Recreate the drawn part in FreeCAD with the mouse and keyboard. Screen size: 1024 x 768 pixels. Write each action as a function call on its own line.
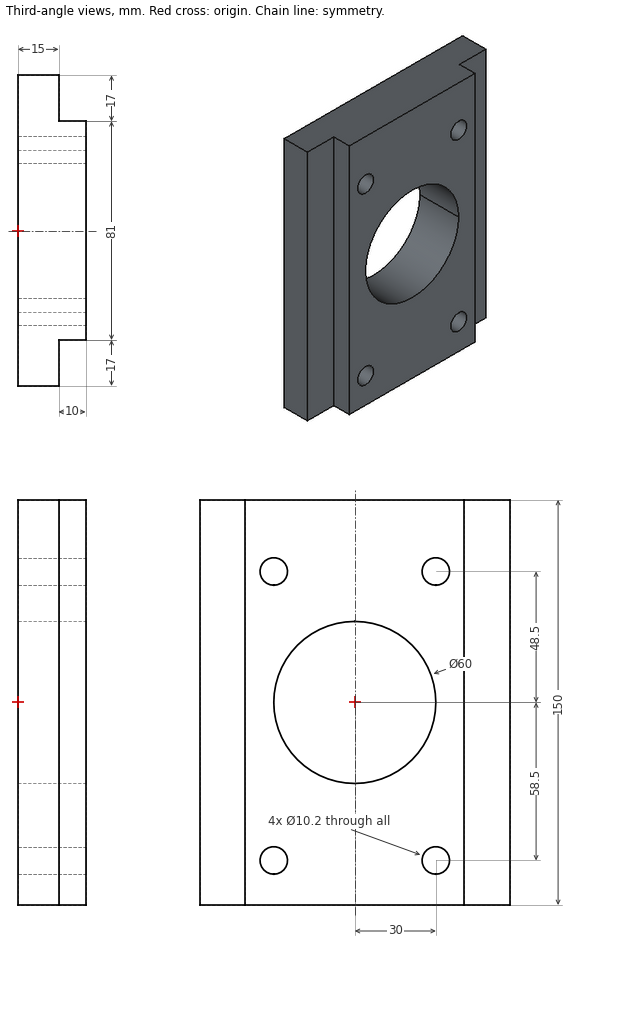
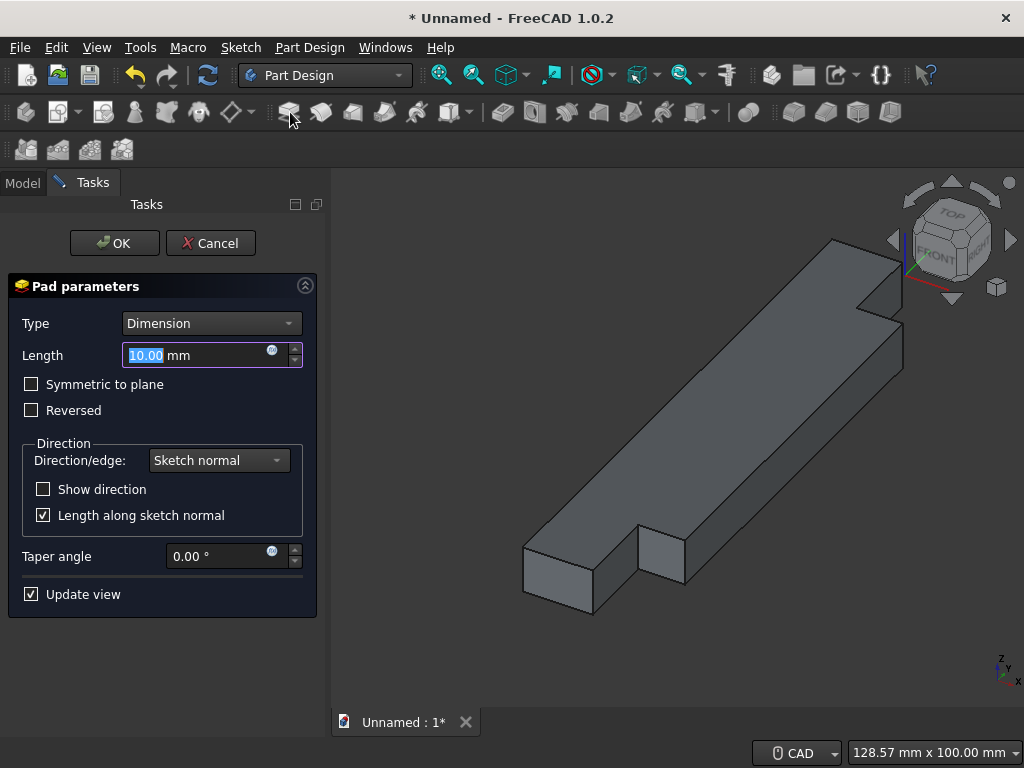
text(150)
key(Tab)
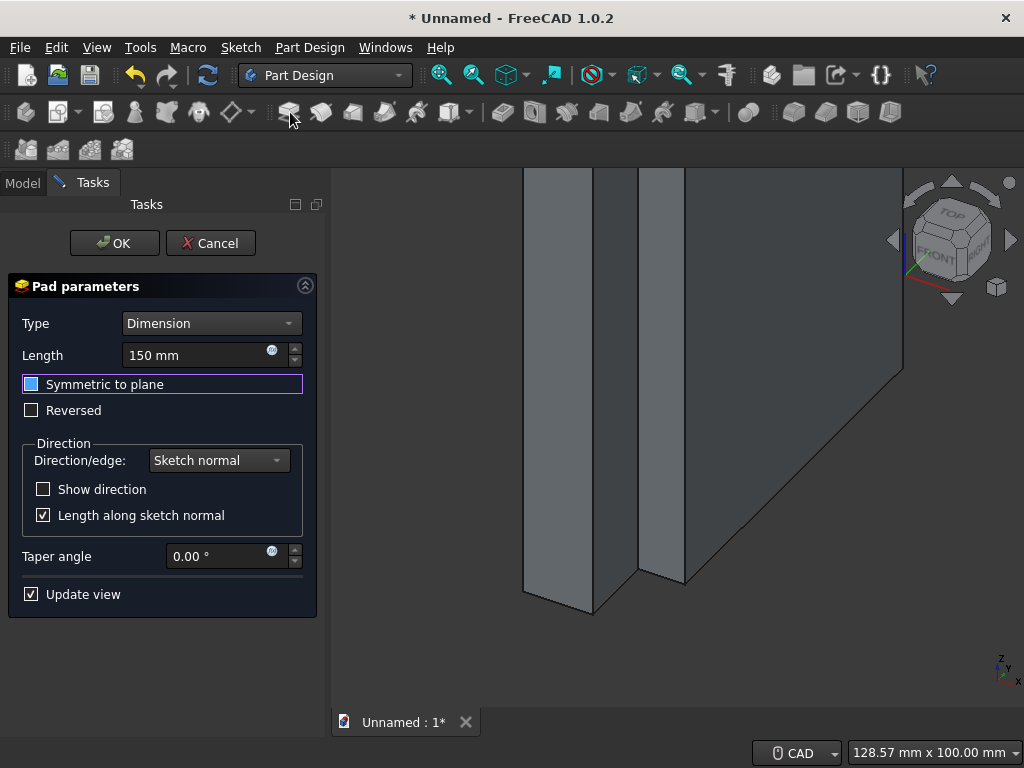
click(30, 384)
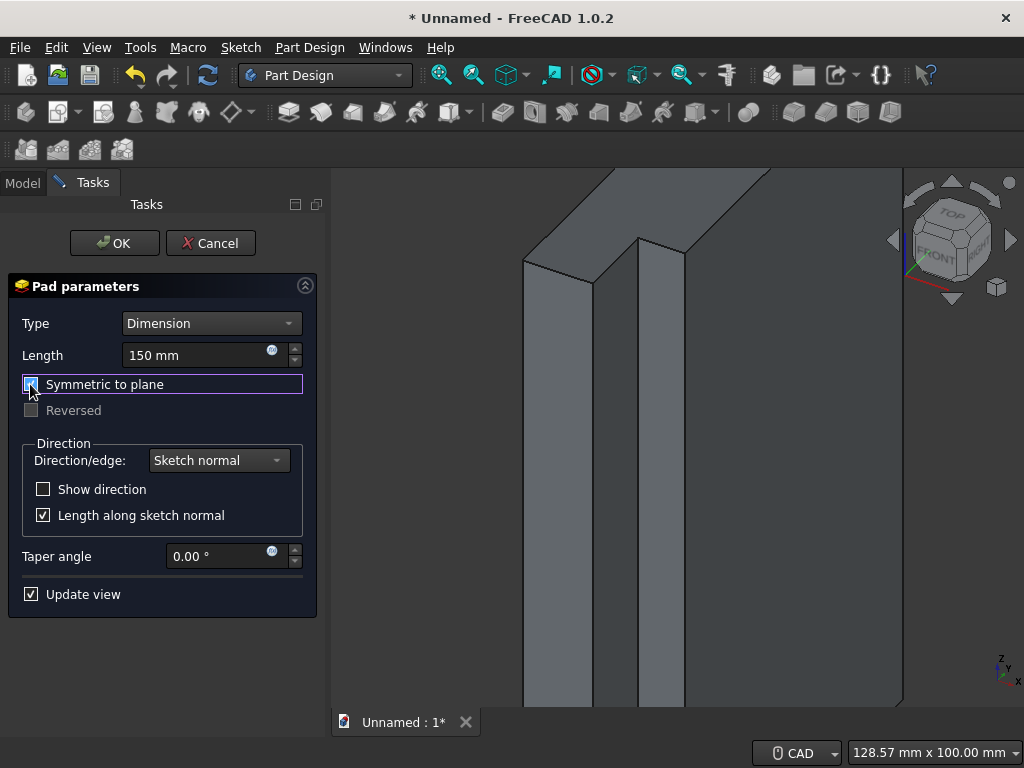
click(115, 243)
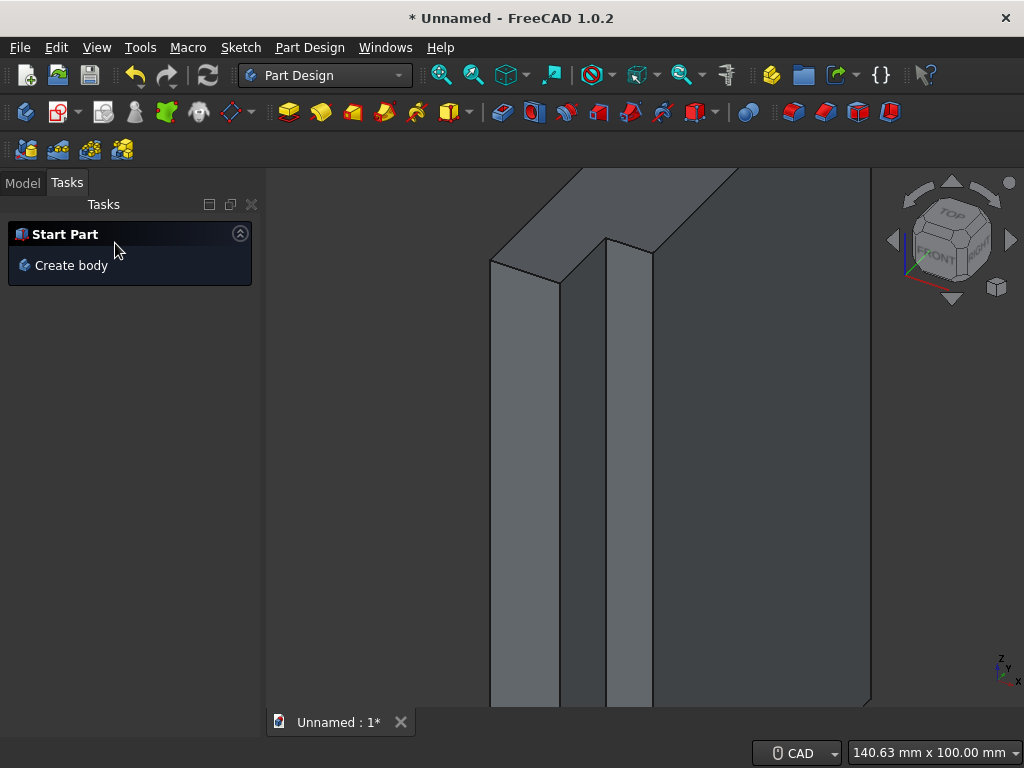
click(442, 76)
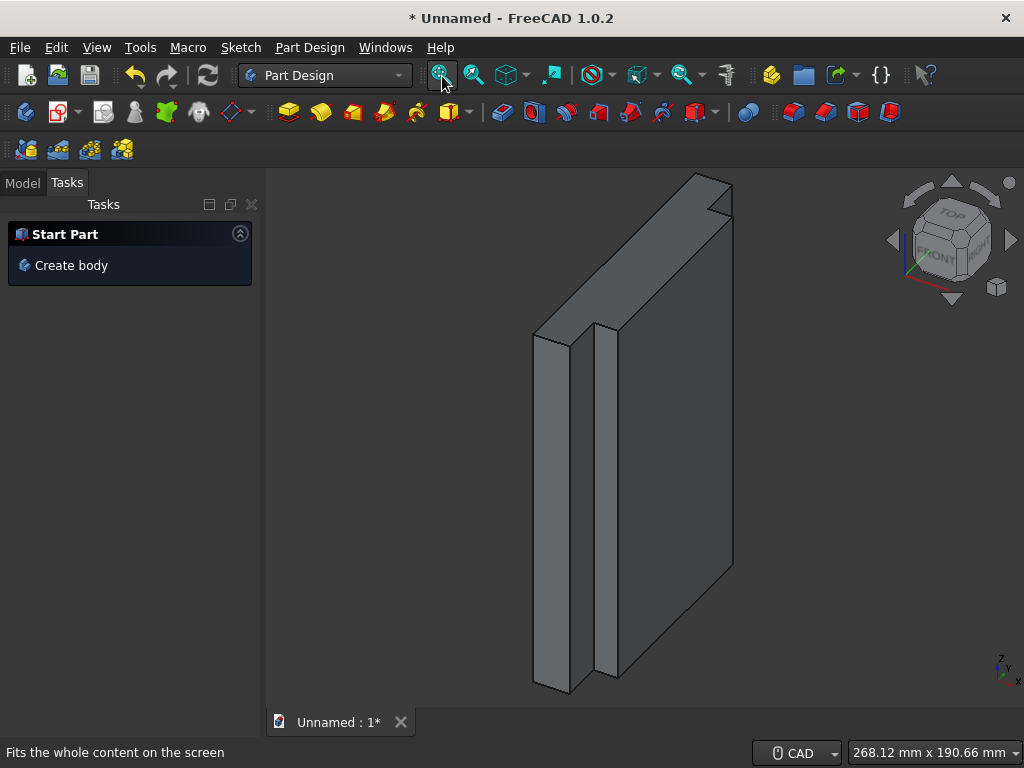
click(58, 112)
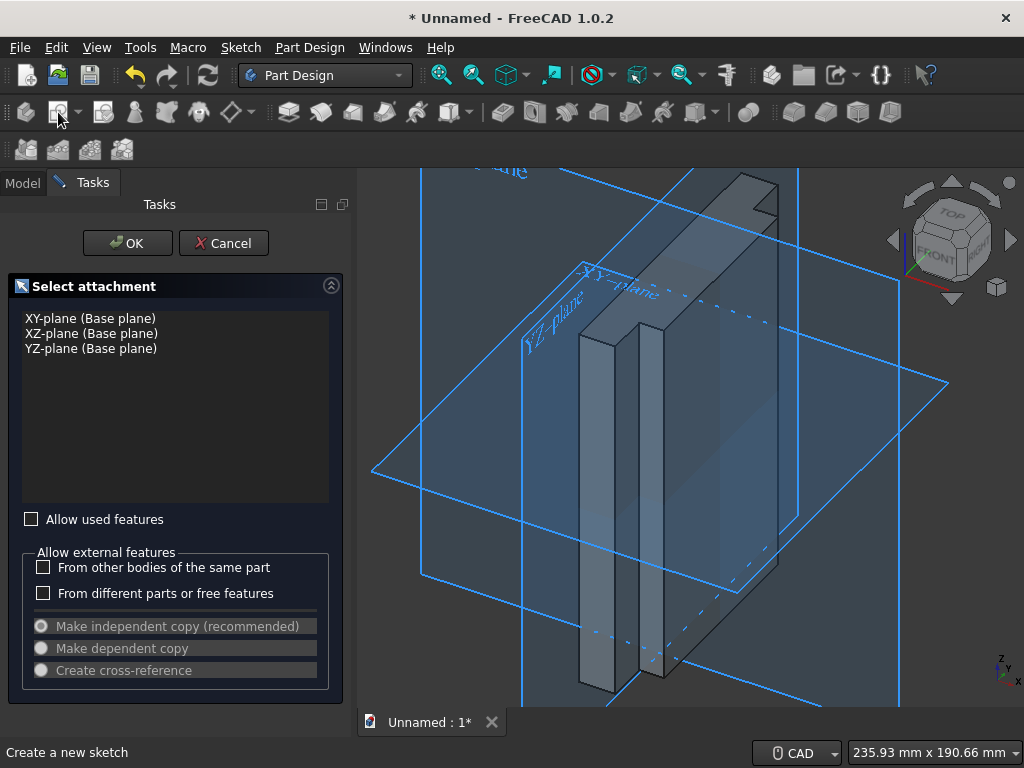
click(82, 348)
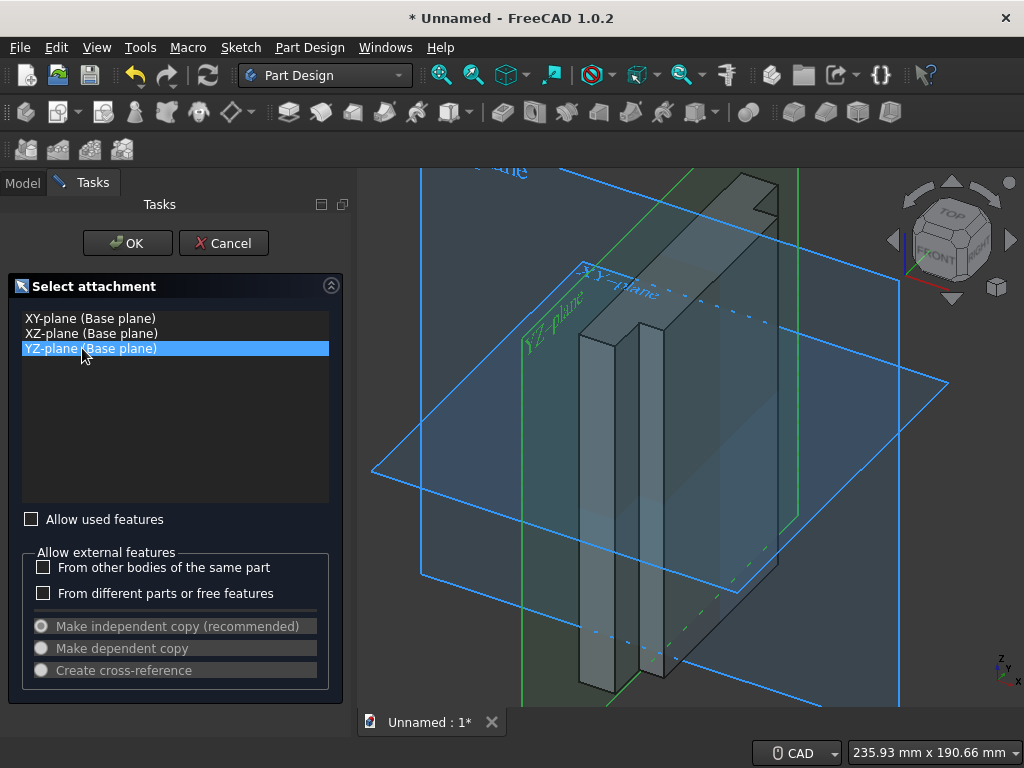
click(128, 243)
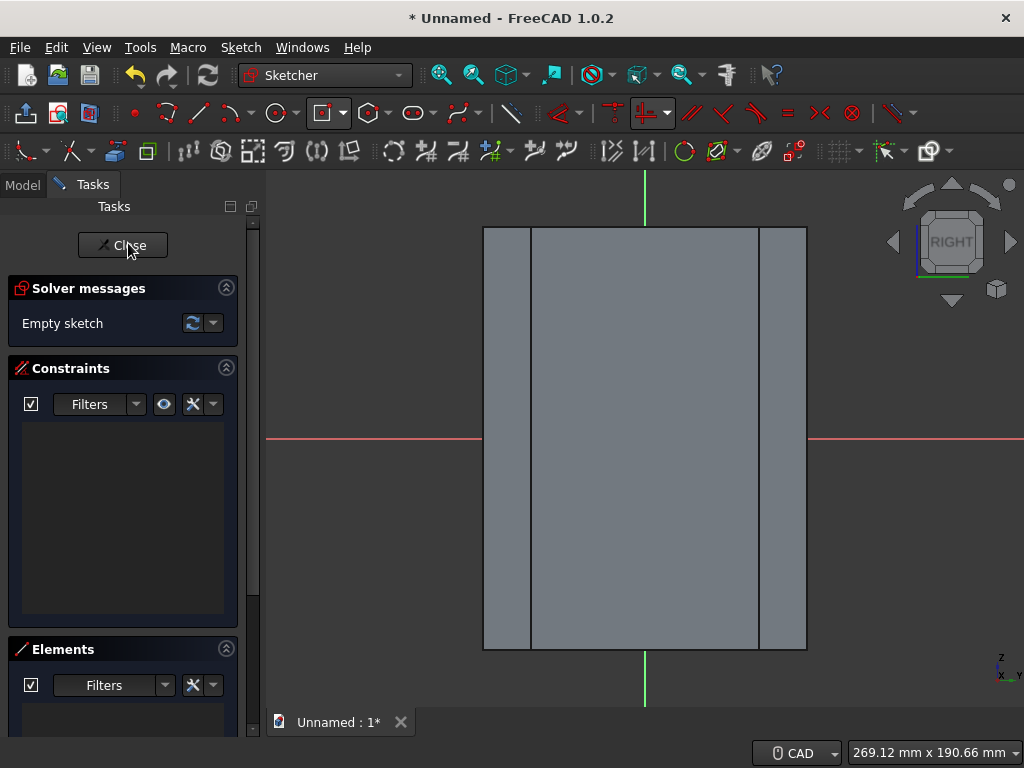
click(90, 114)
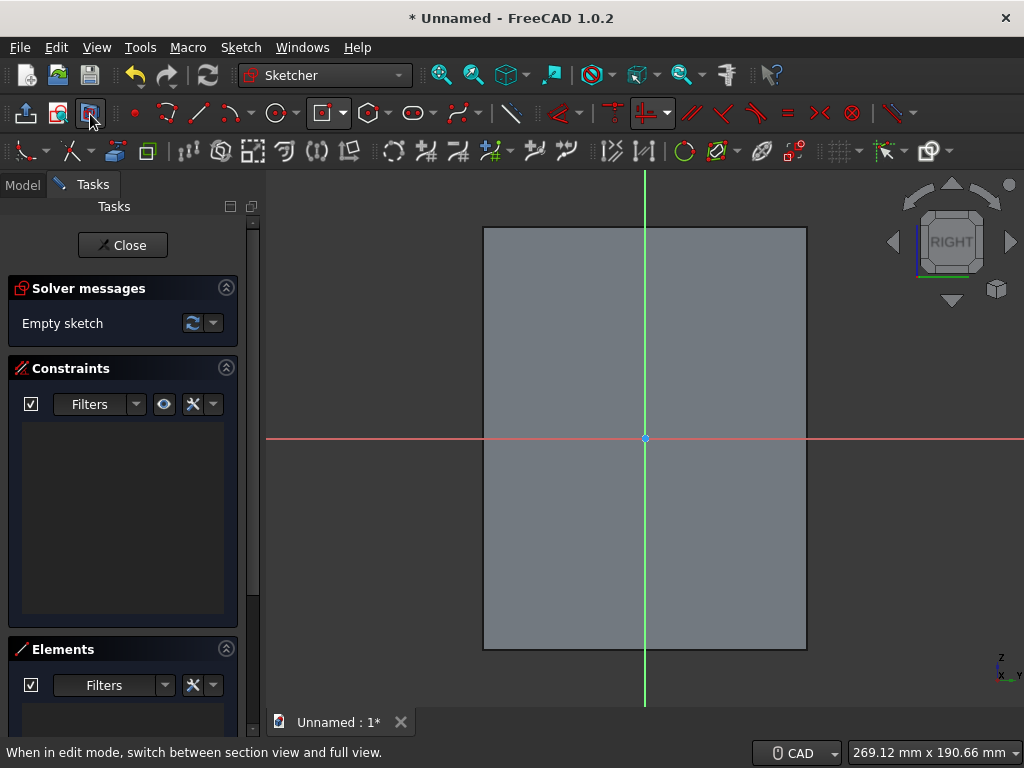
scroll(728, 438, up, 3)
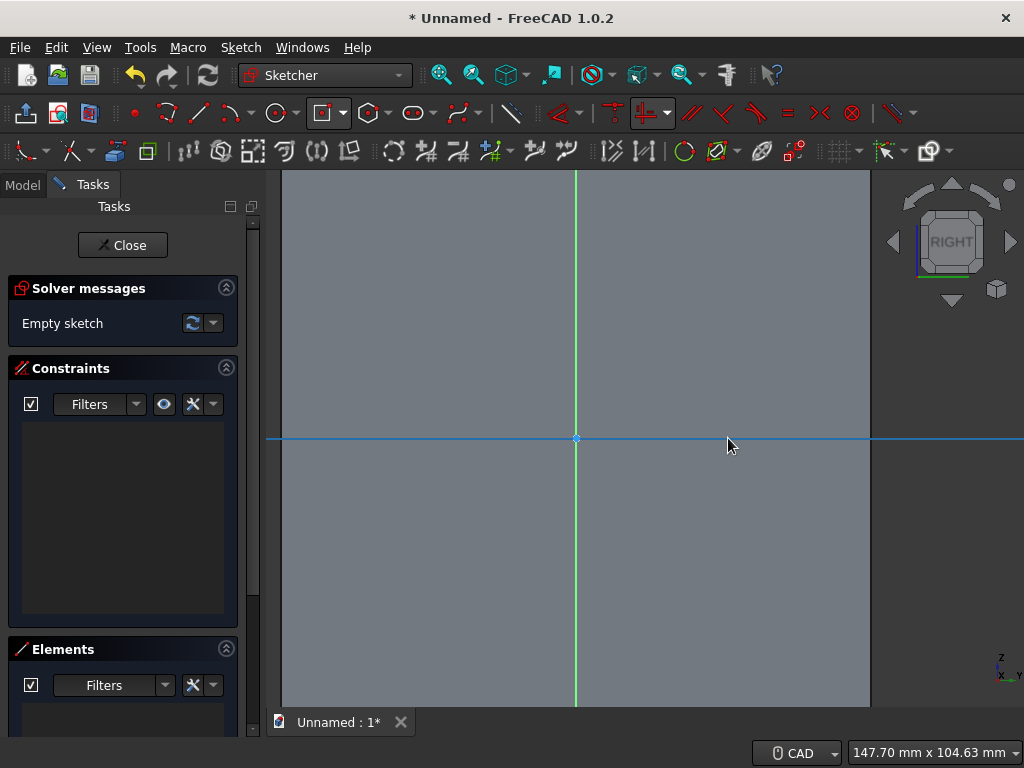
click(276, 114)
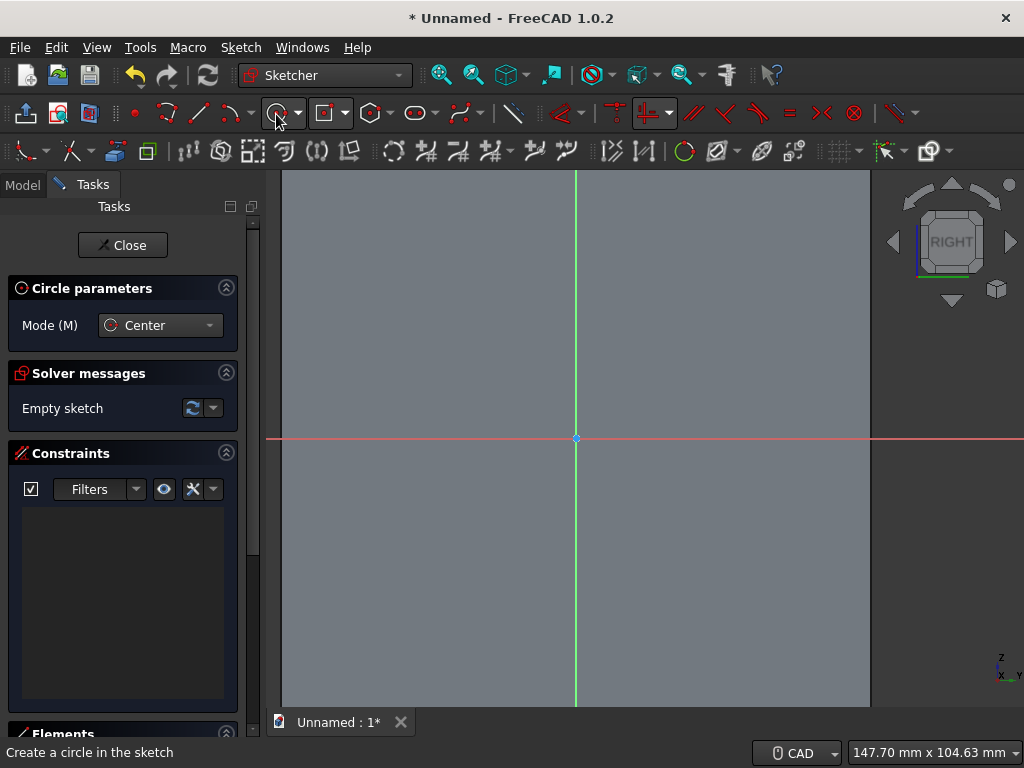
click(576, 438)
click(685, 330)
key(Escape)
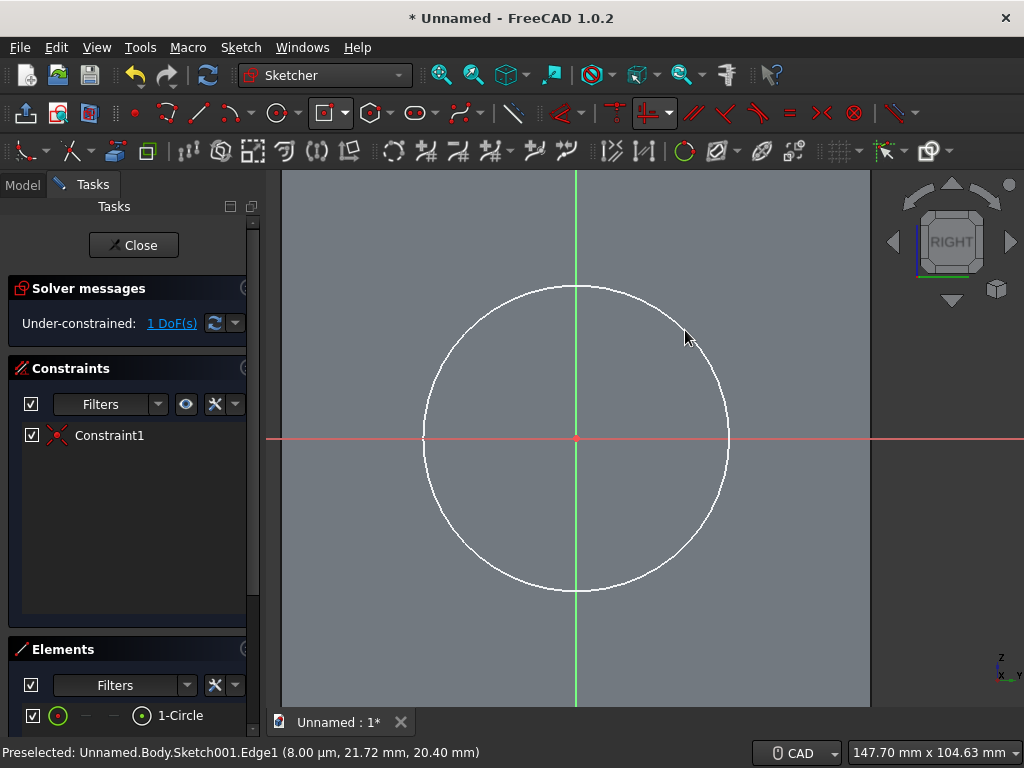
click(560, 114)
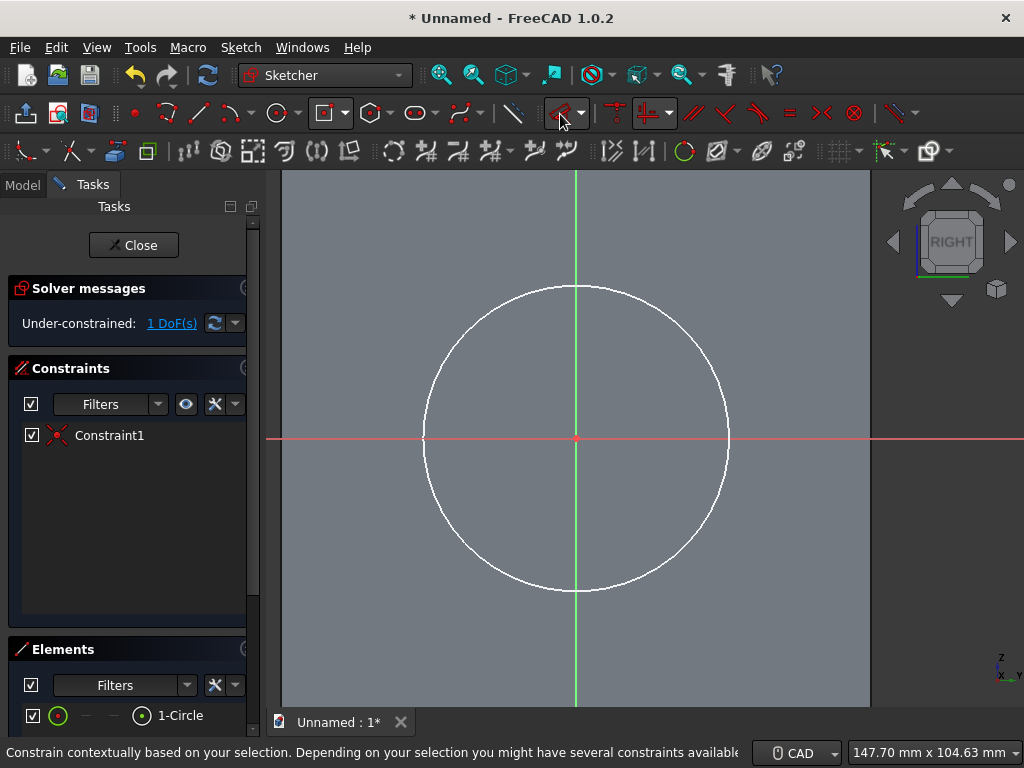
click(684, 330)
click(707, 307)